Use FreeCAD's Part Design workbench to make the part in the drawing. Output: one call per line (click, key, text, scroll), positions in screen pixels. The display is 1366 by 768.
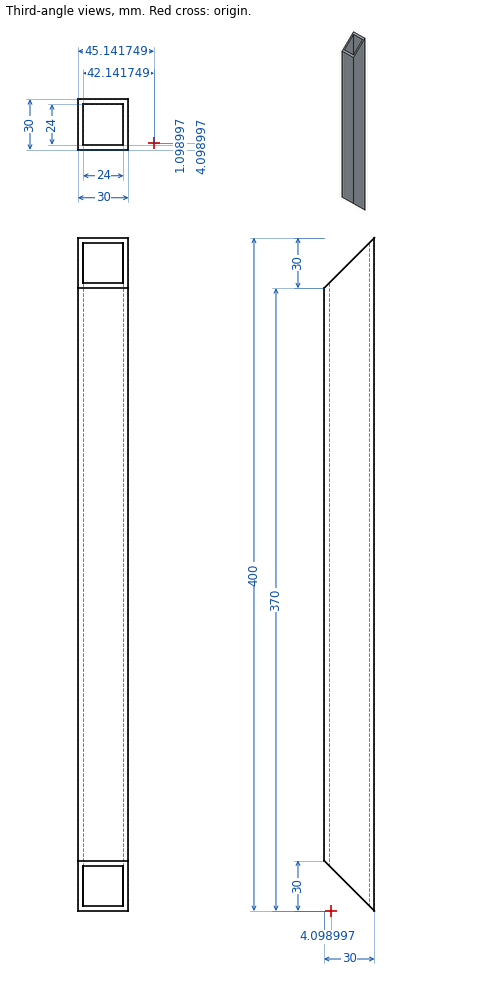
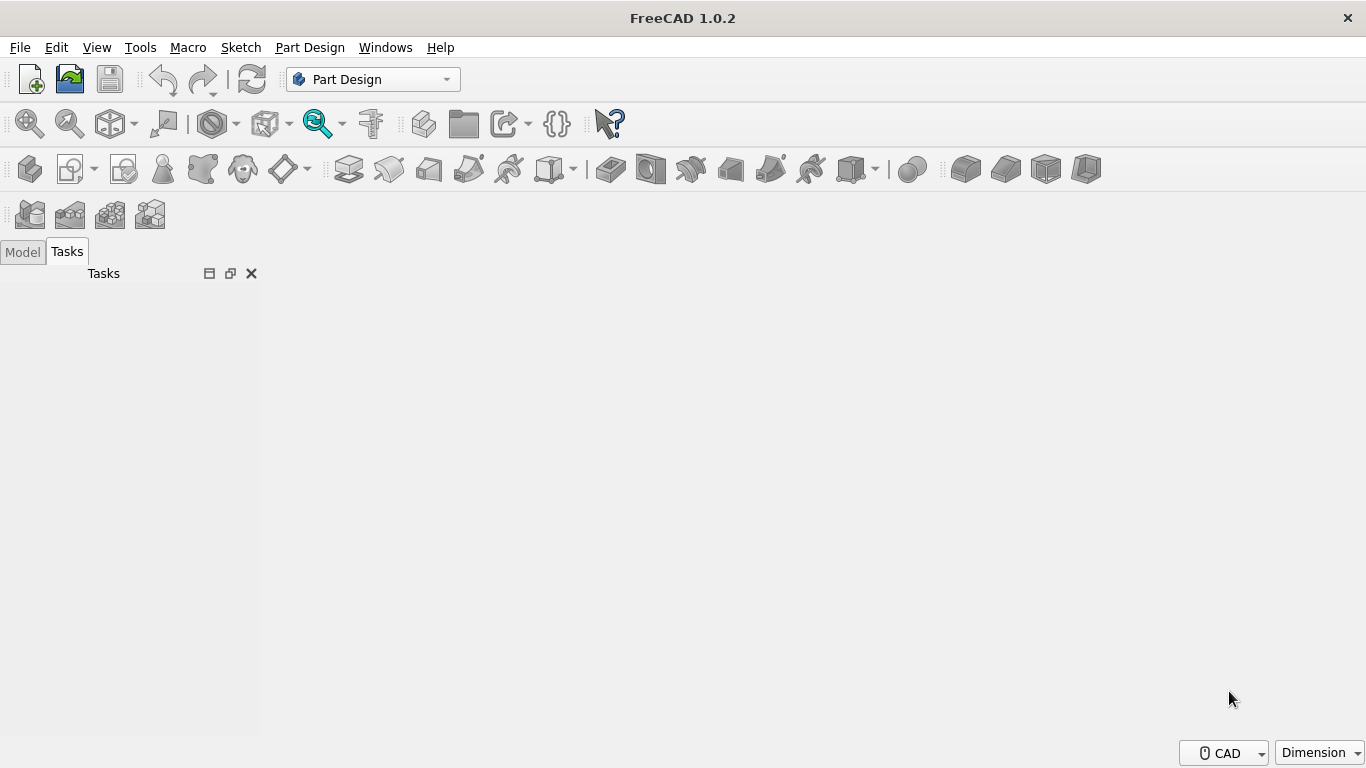
click(30, 80)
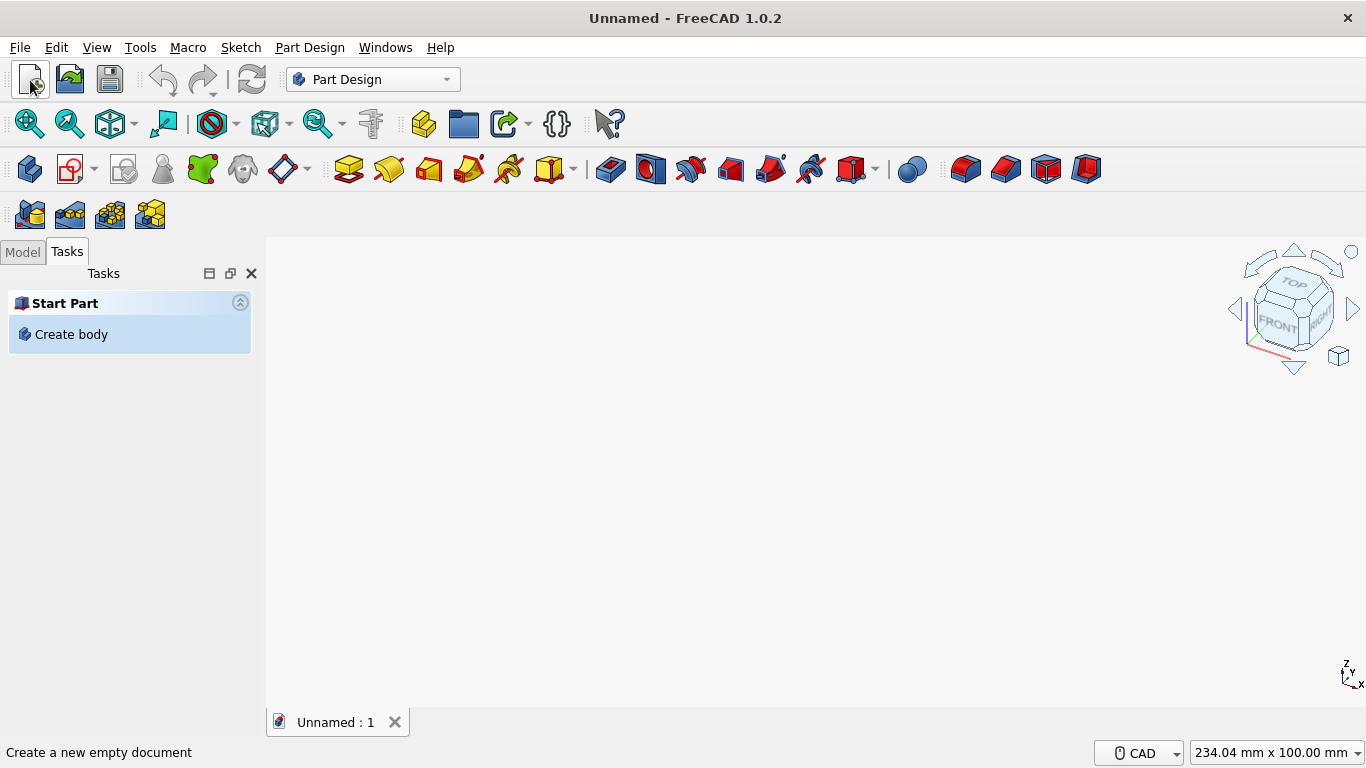
click(70, 170)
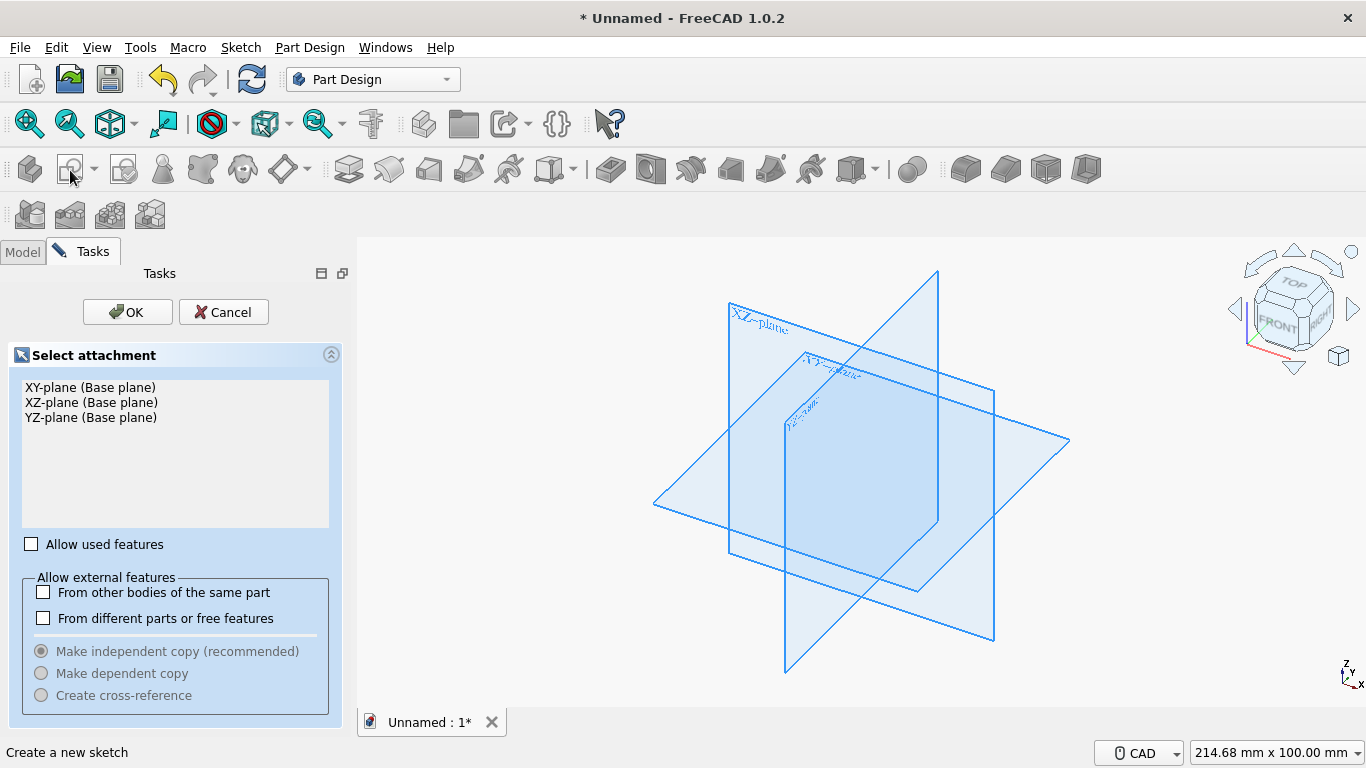
click(82, 388)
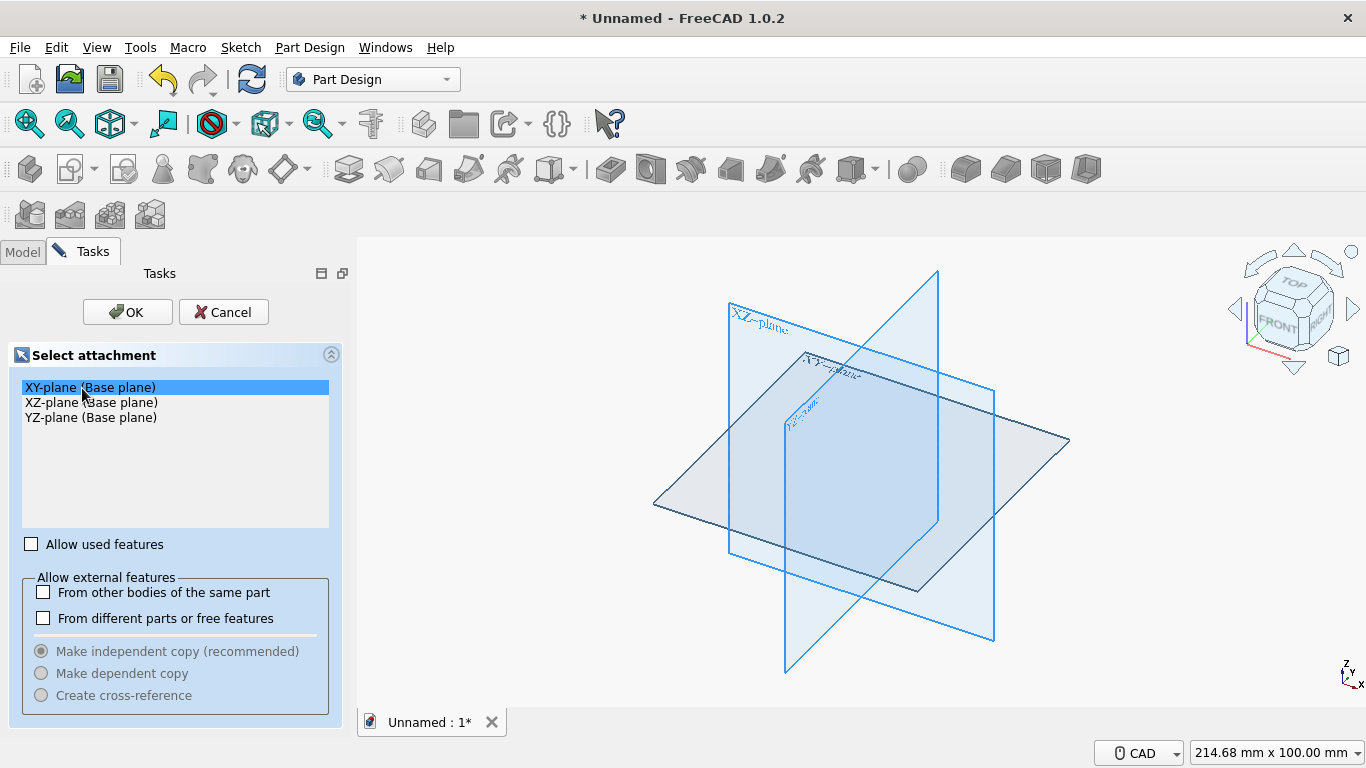
click(128, 312)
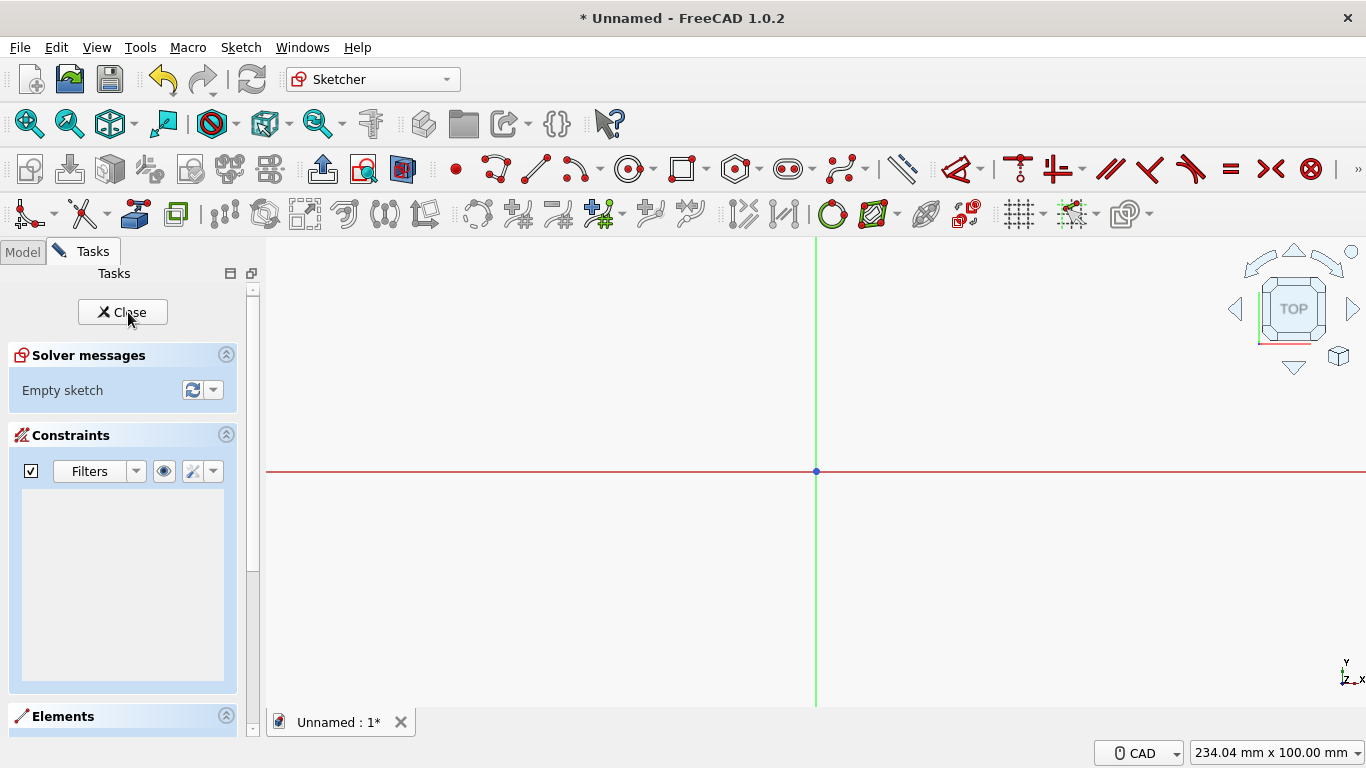
scroll(679, 379, up, 4)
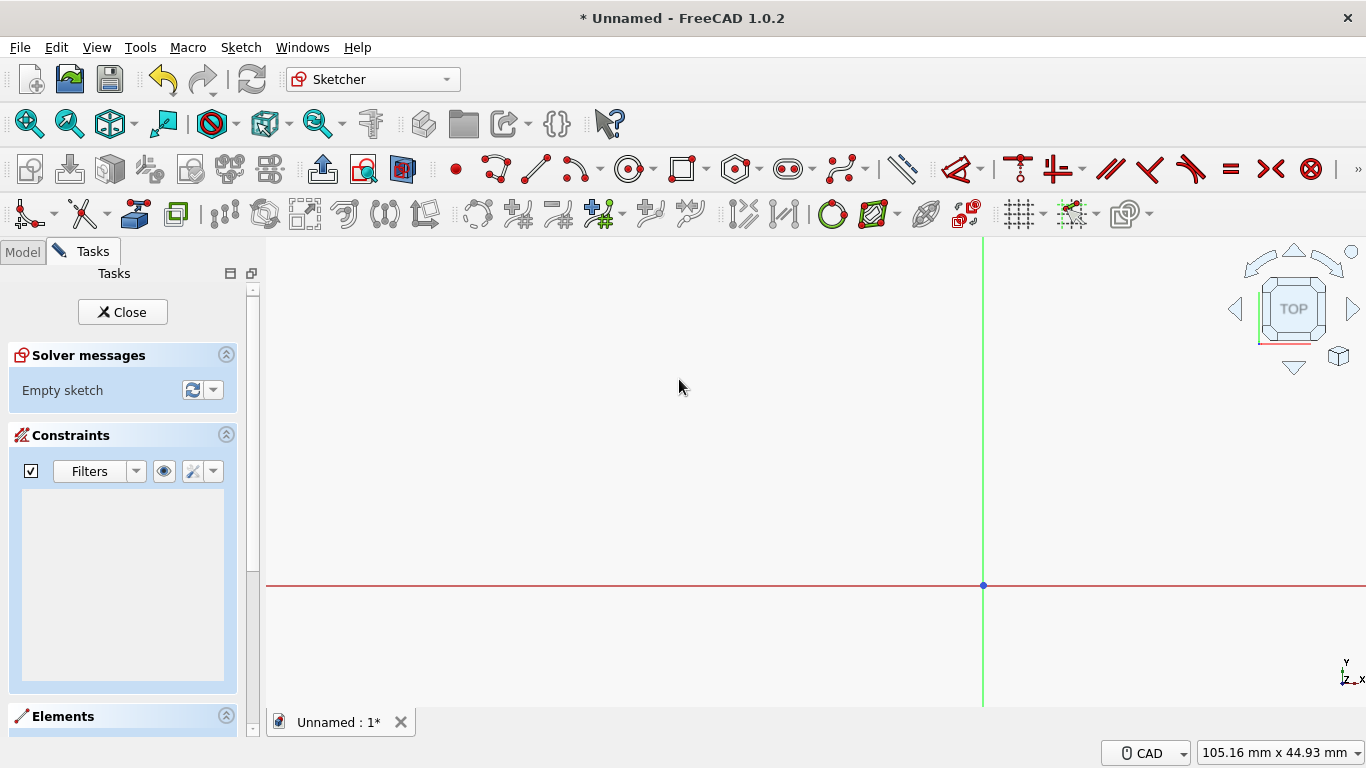
click(682, 170)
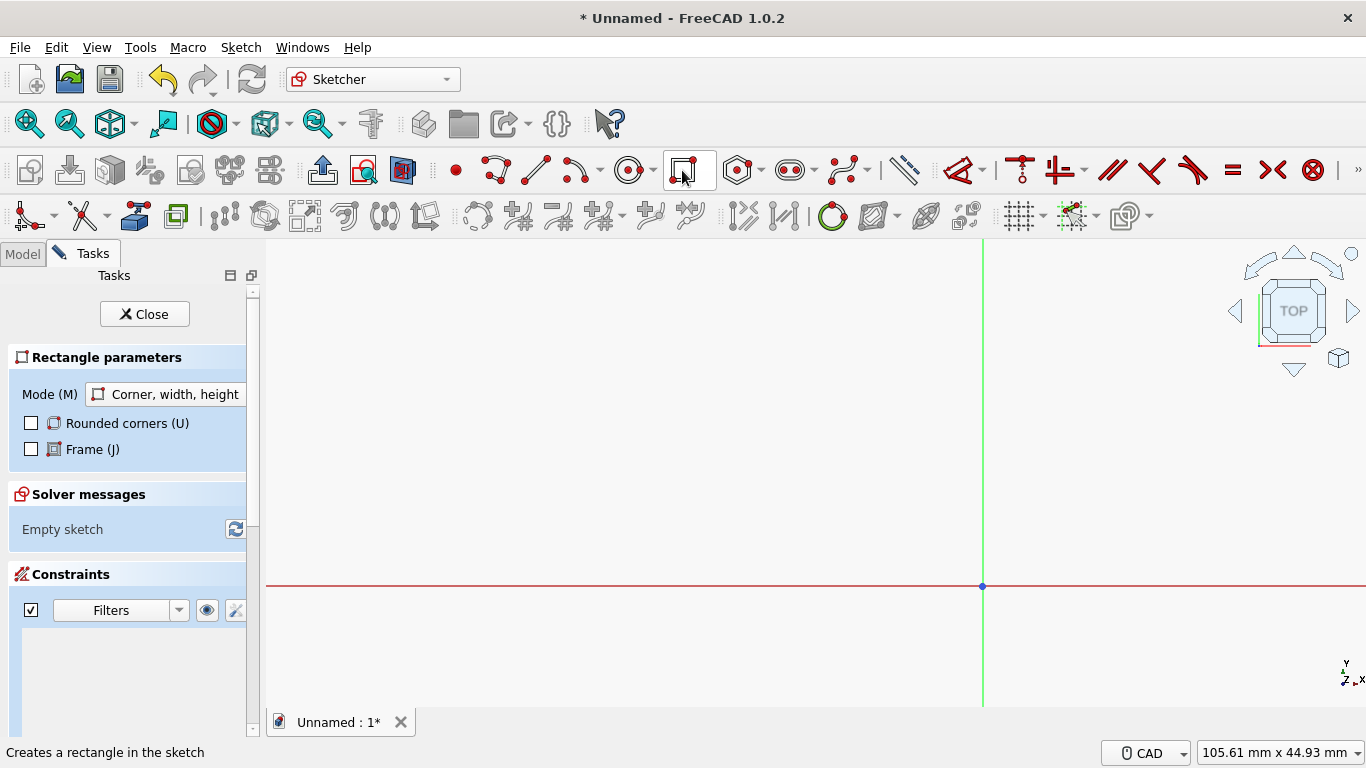
click(513, 316)
click(825, 629)
key(Escape)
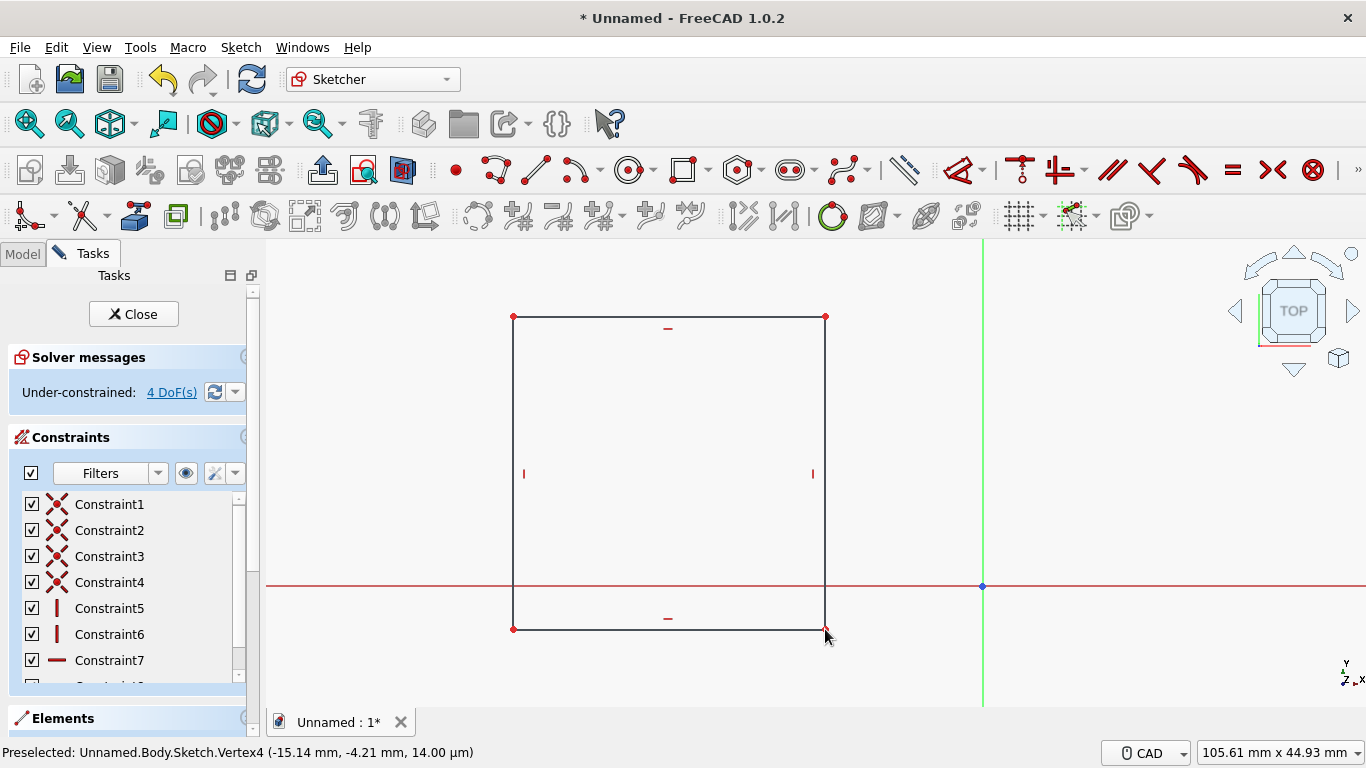
click(958, 170)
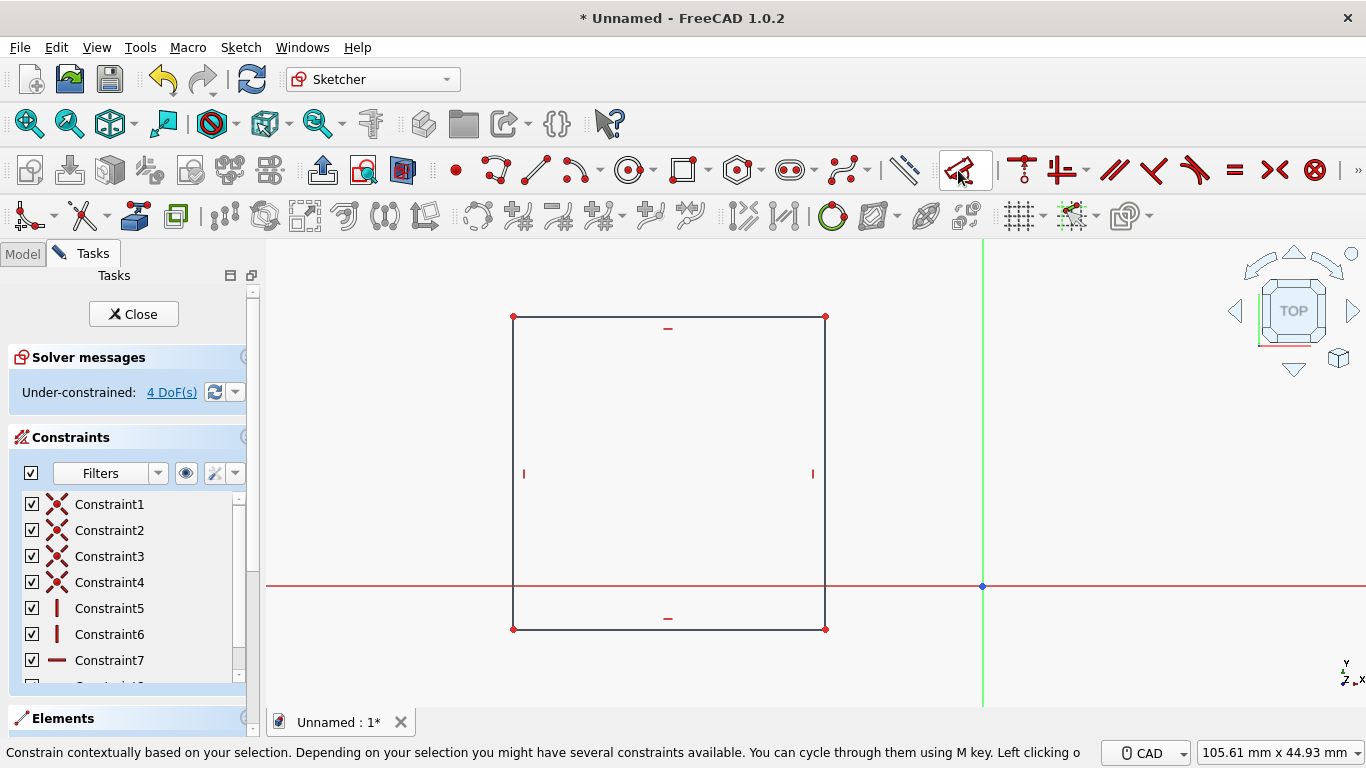
click(513, 411)
click(479, 474)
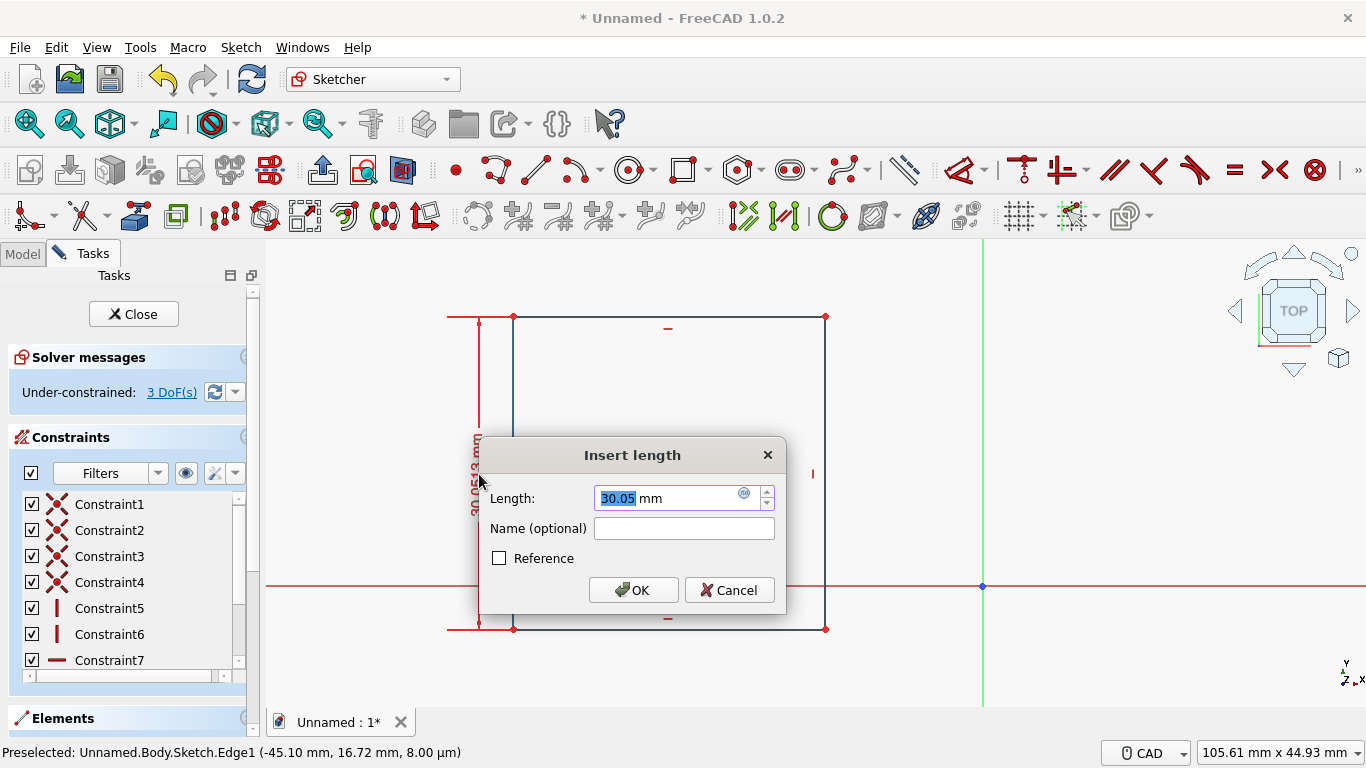
text(30)
key(Return)